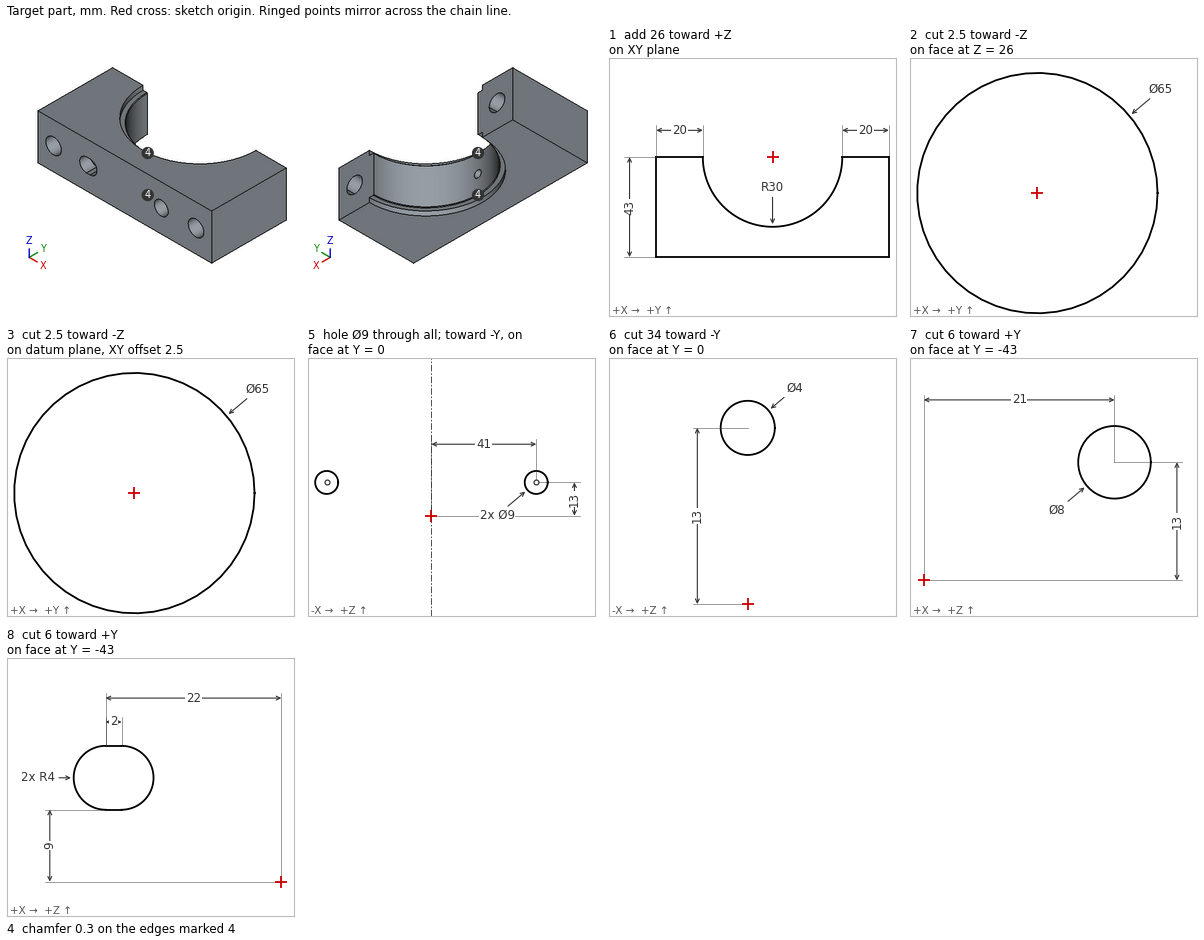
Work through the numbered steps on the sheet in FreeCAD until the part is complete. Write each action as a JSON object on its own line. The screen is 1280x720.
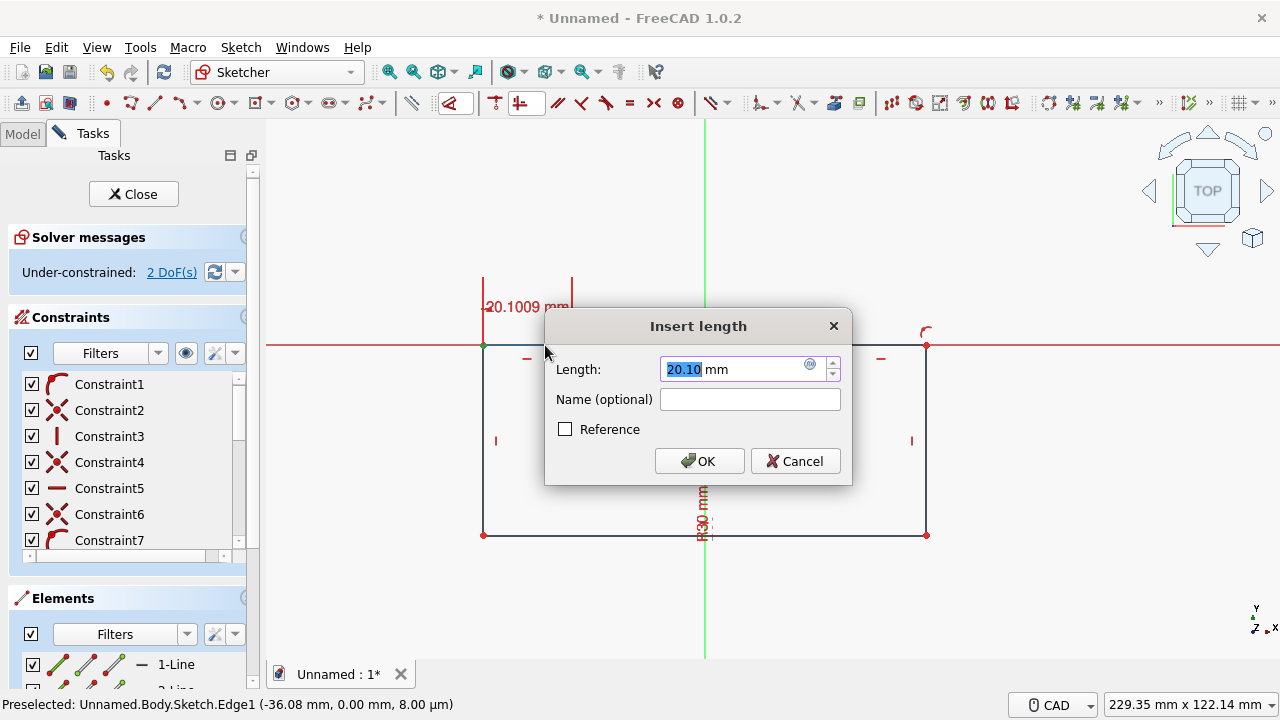
{"action": "type", "text": "20"}
{"action": "key", "text": "Return"}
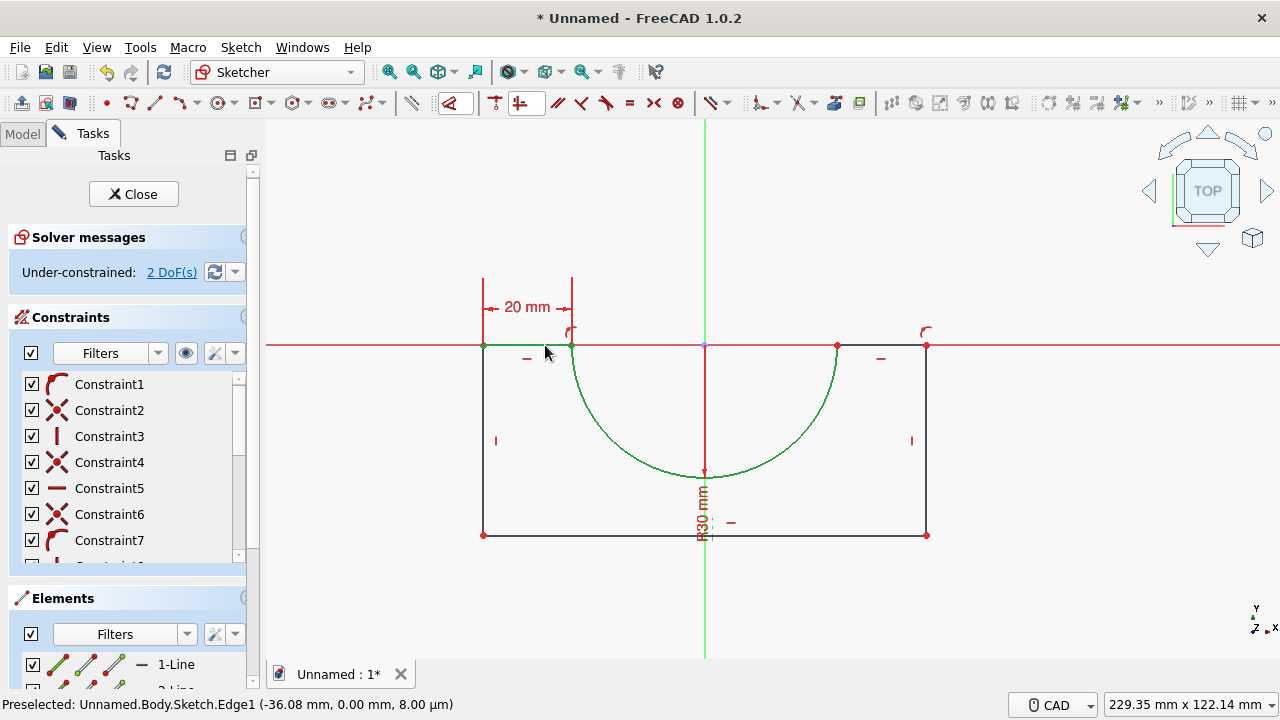
{"action": "left_click", "coordinate": [483, 402]}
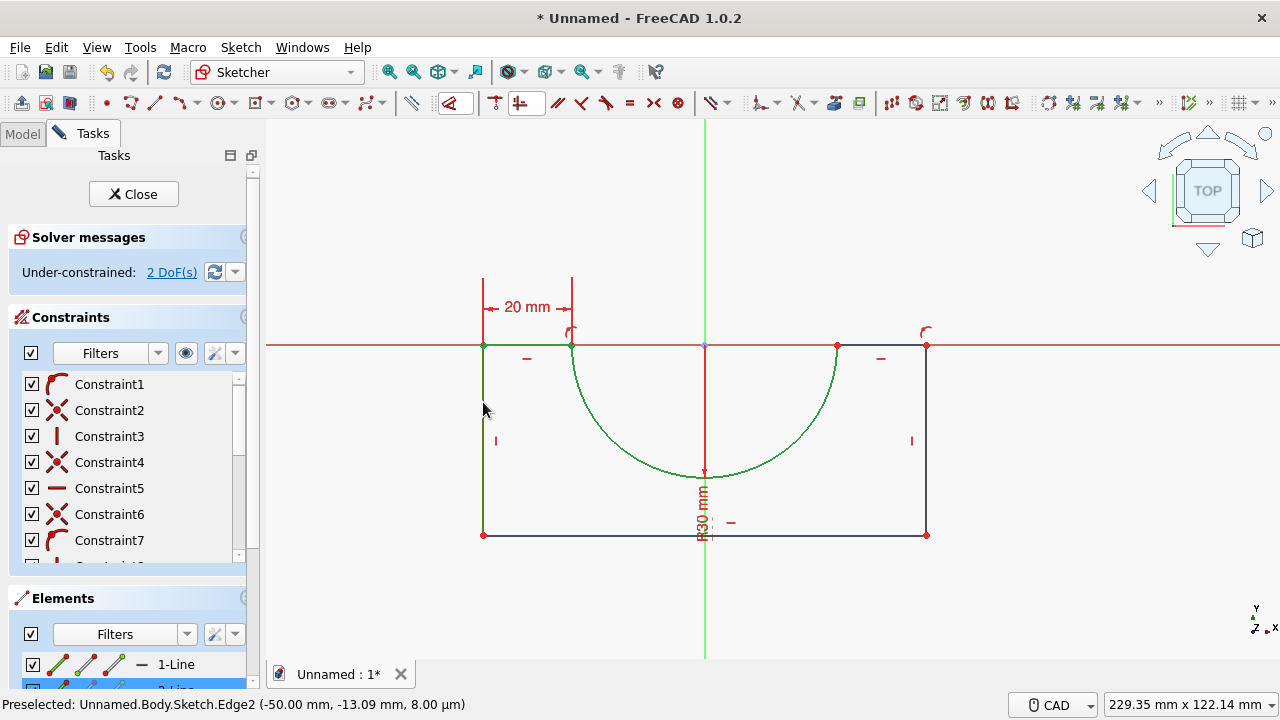
{"action": "left_click", "coordinate": [468, 104]}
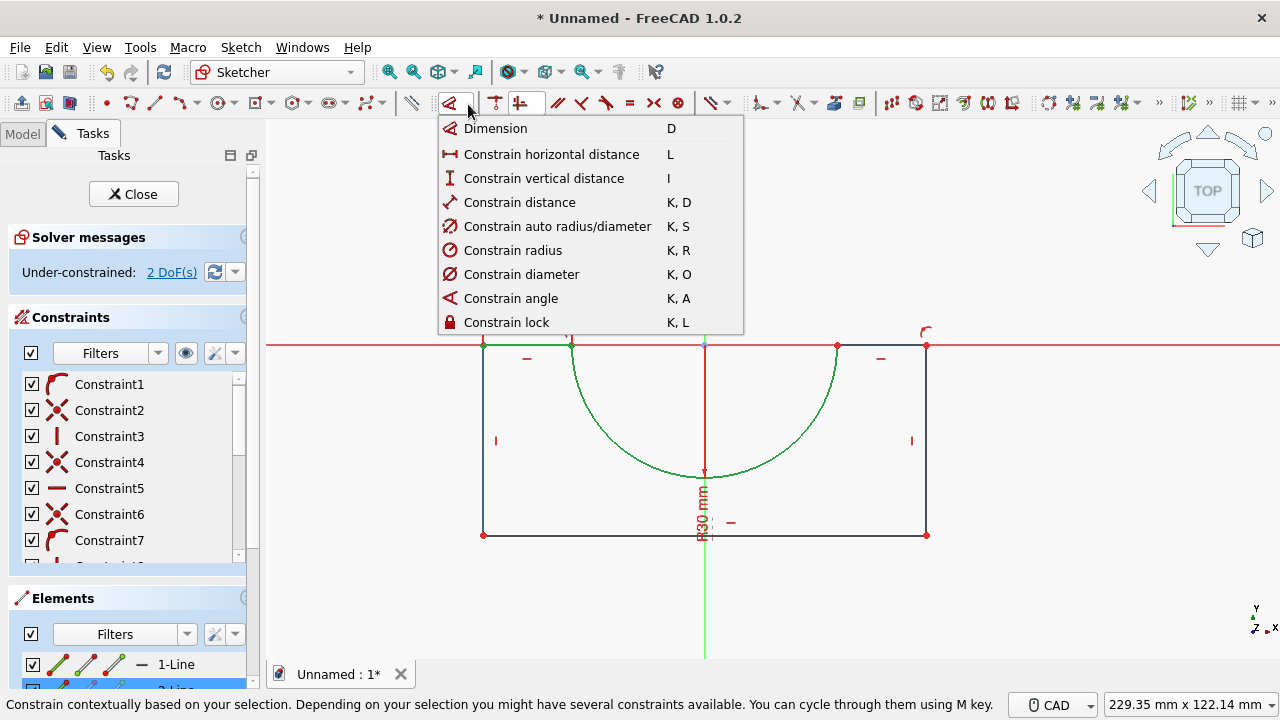
{"action": "left_click", "coordinate": [591, 178]}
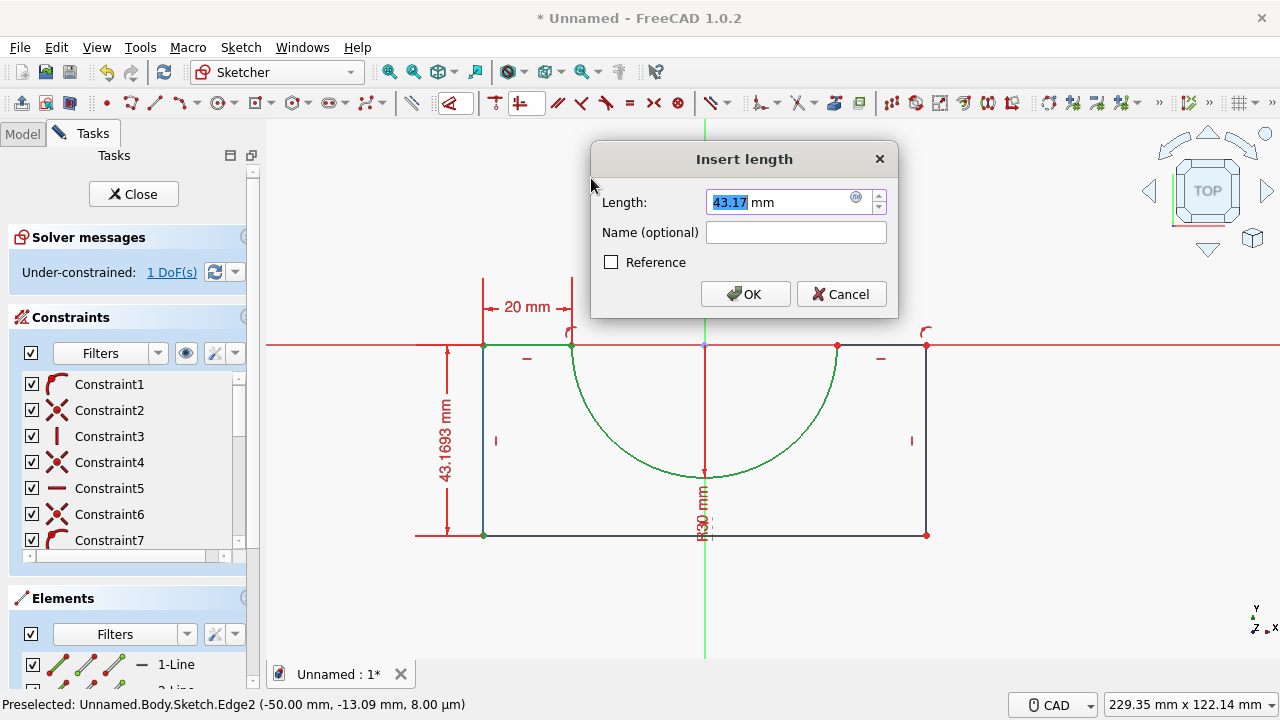
{"action": "type", "text": "43"}
{"action": "key", "text": "Return"}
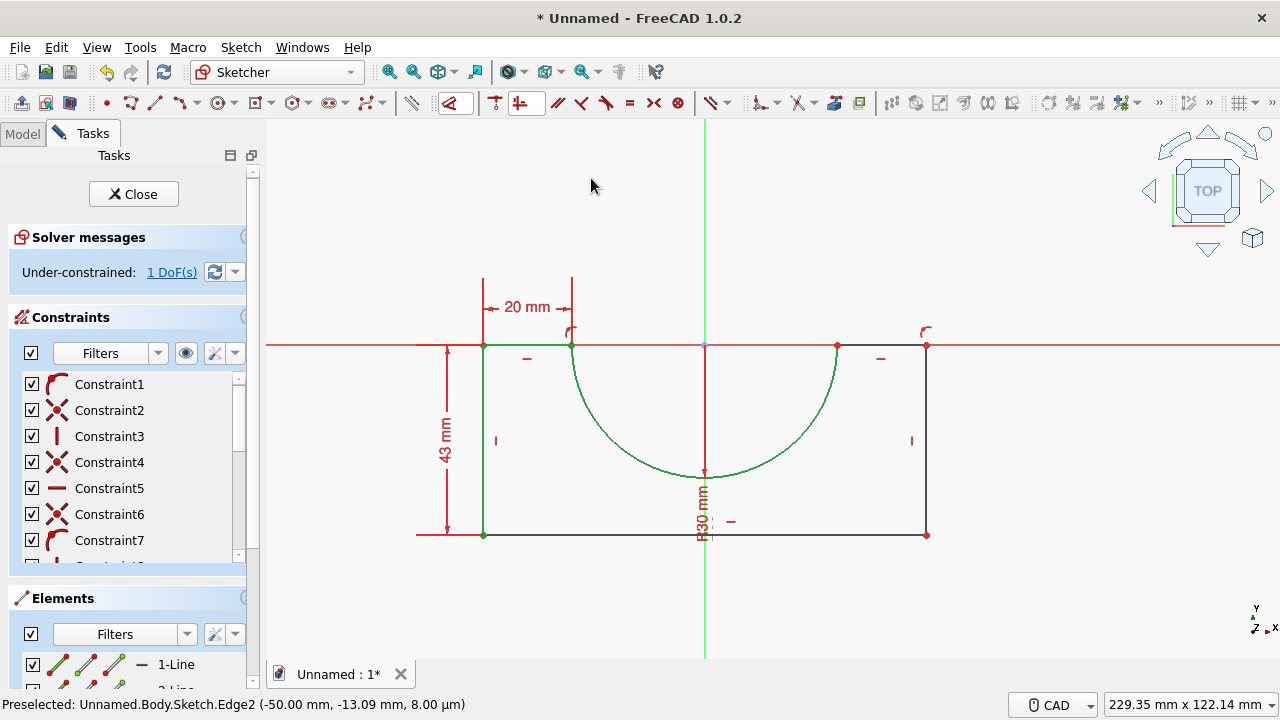
{"action": "left_click", "coordinate": [899, 345]}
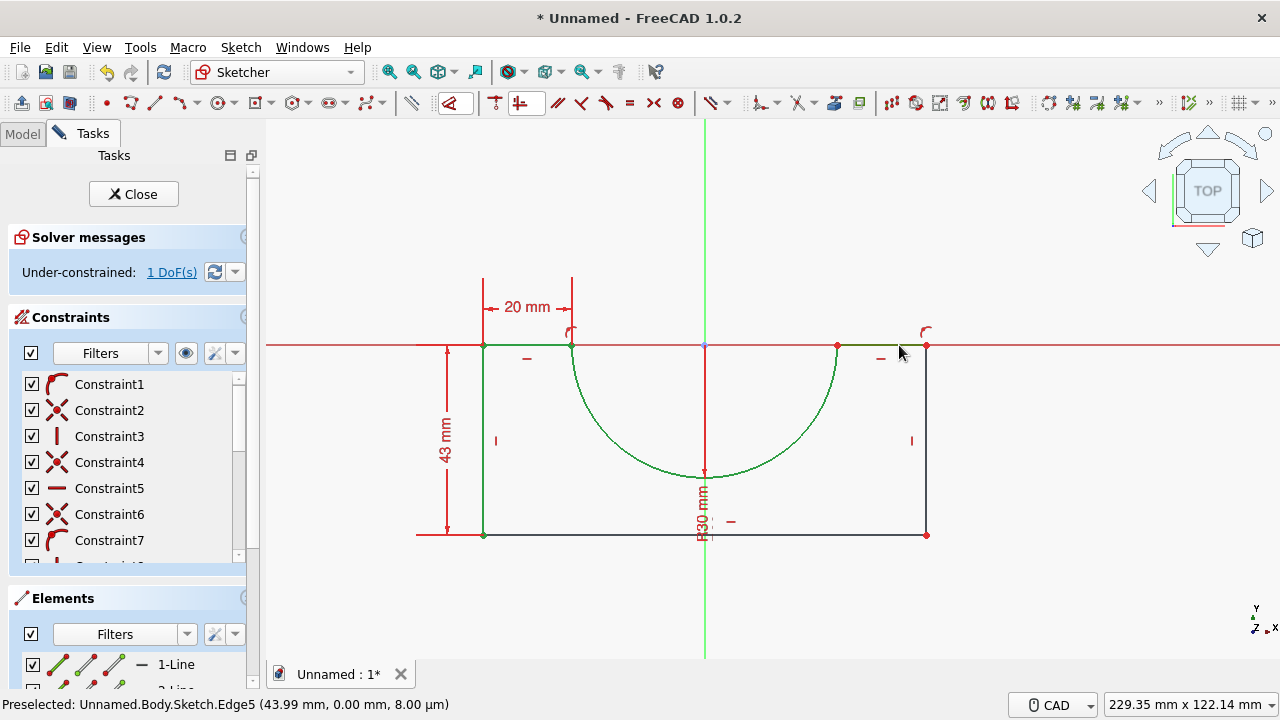
{"action": "left_click", "coordinate": [468, 104]}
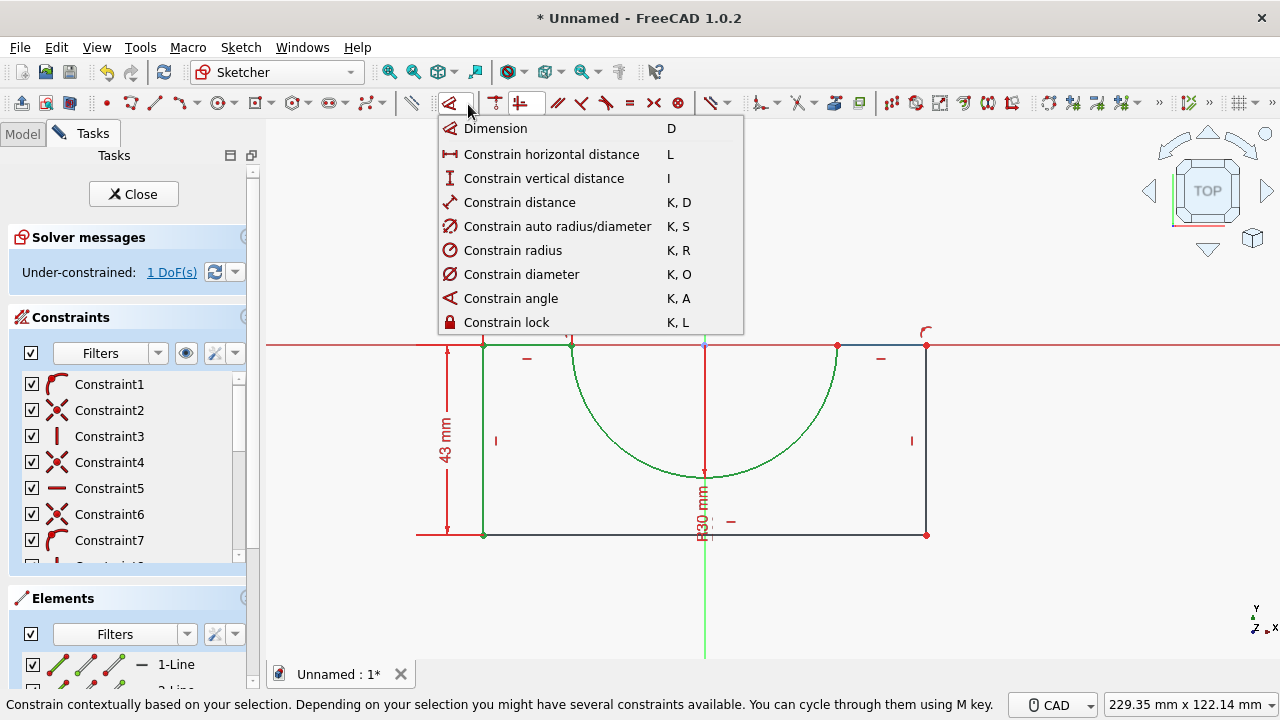
{"action": "left_click", "coordinate": [591, 154]}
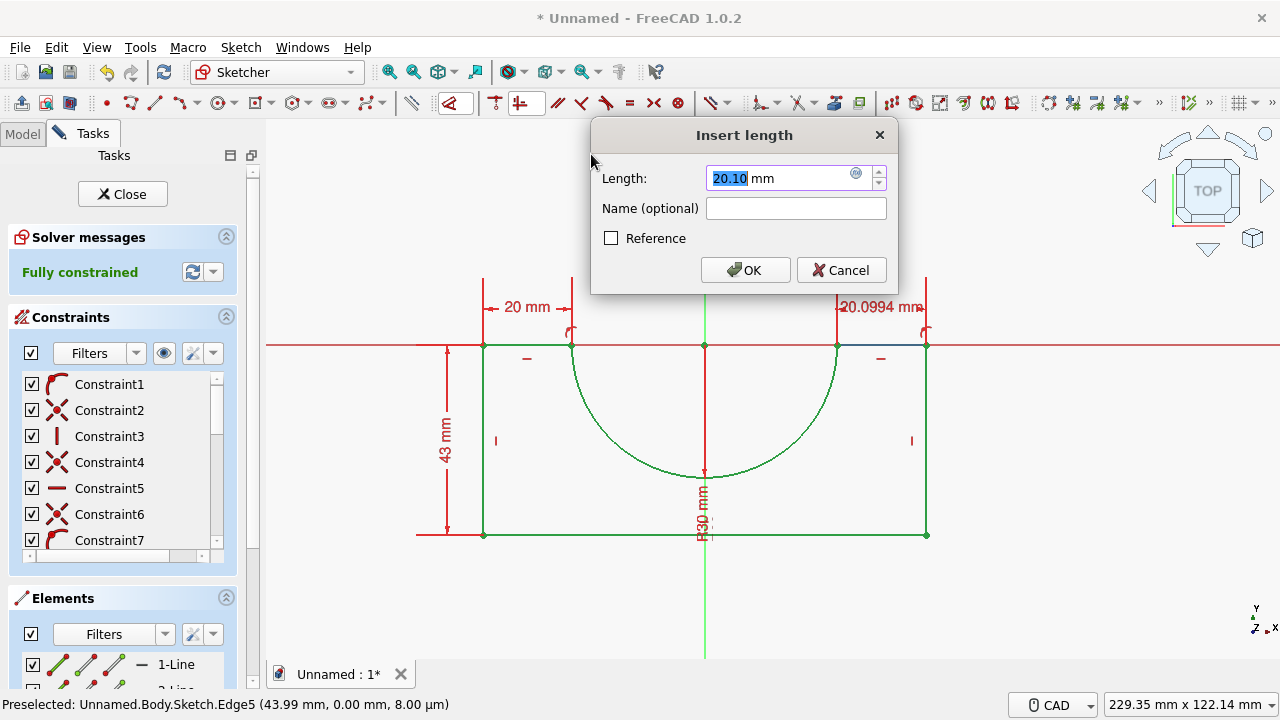
{"action": "type", "text": "20"}
{"action": "key", "text": "Return"}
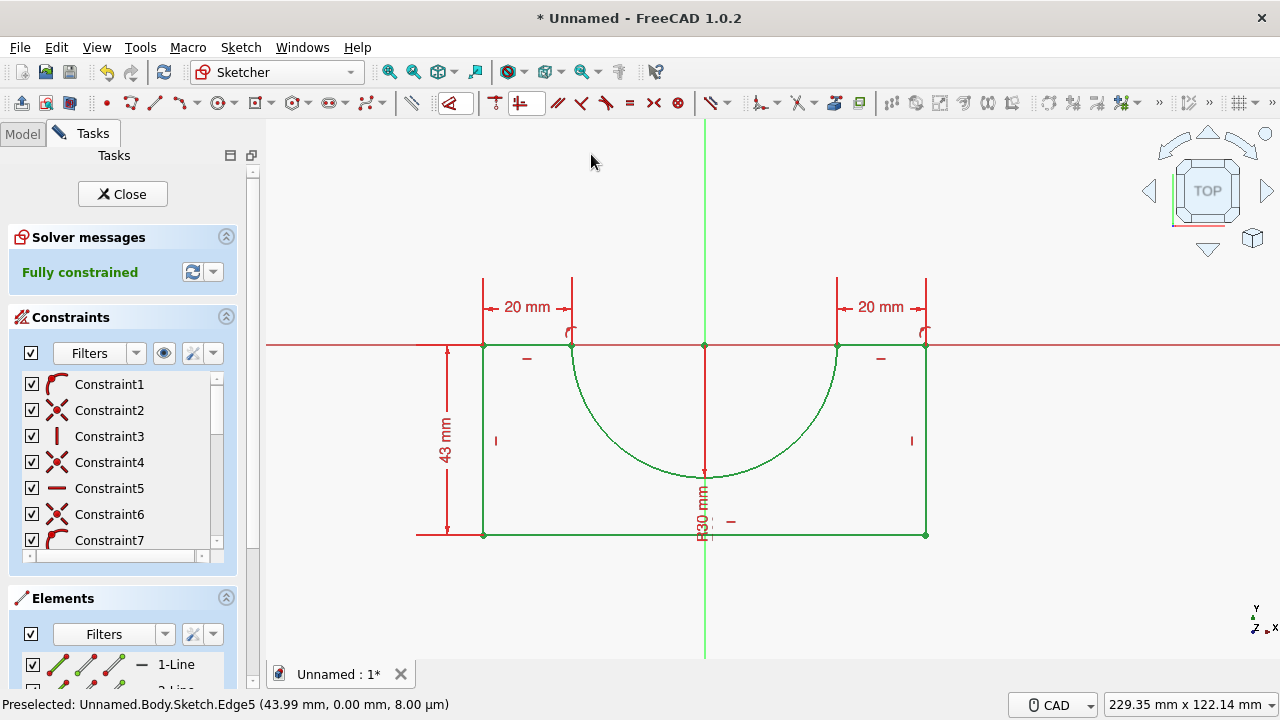
{"action": "left_click", "coordinate": [123, 194]}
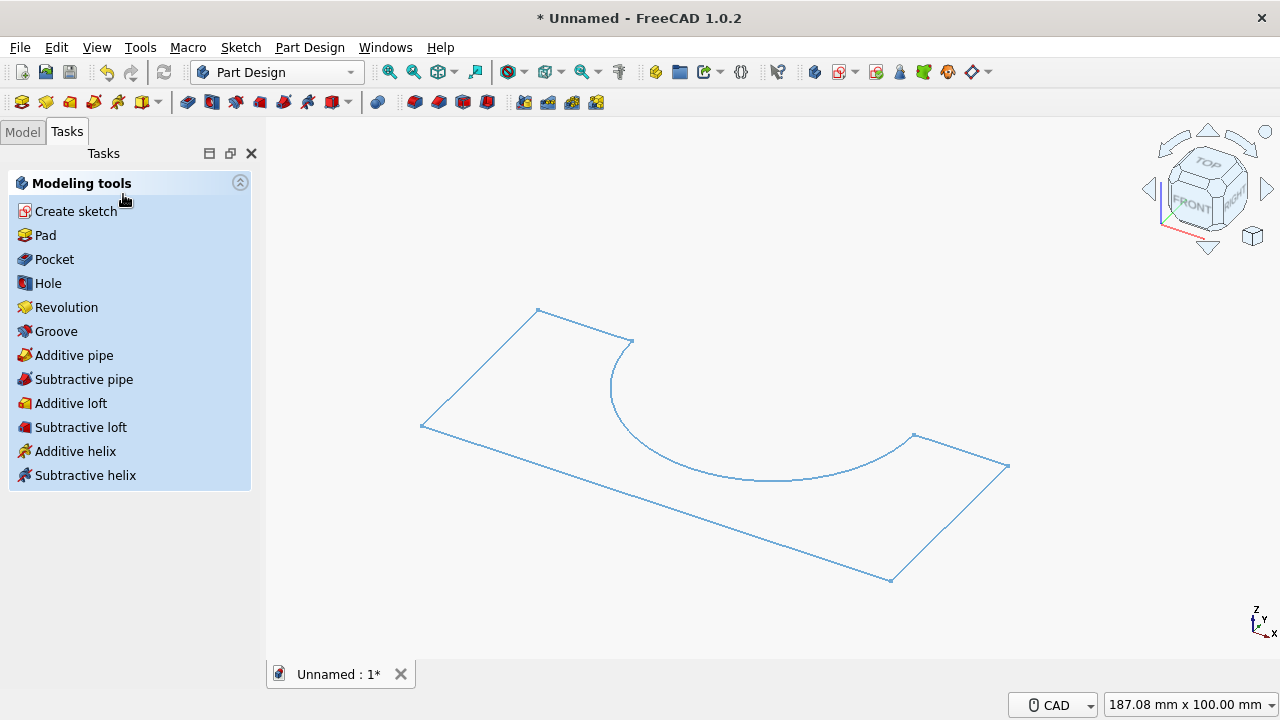
{"action": "left_click", "coordinate": [22, 102]}